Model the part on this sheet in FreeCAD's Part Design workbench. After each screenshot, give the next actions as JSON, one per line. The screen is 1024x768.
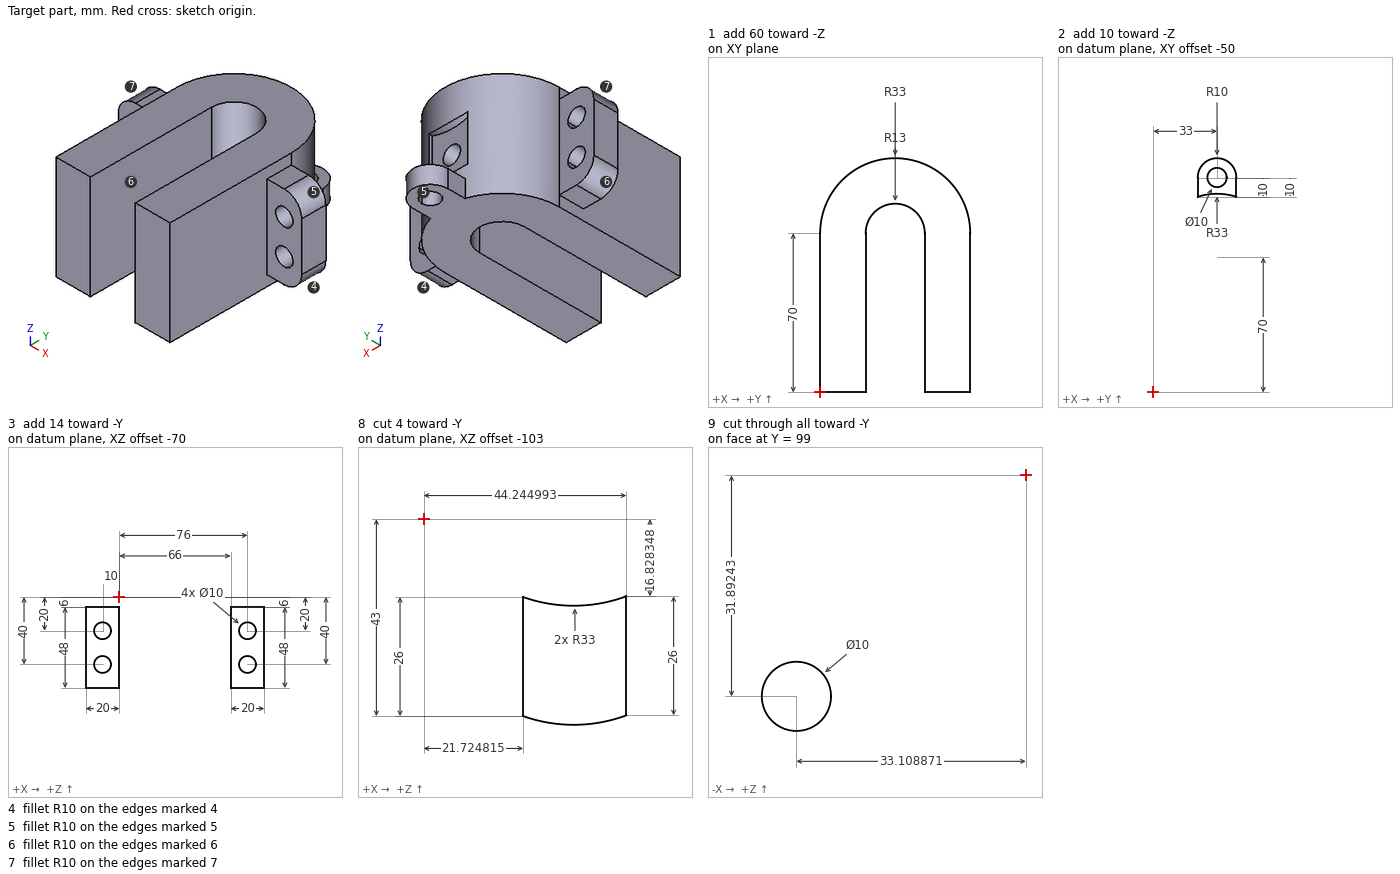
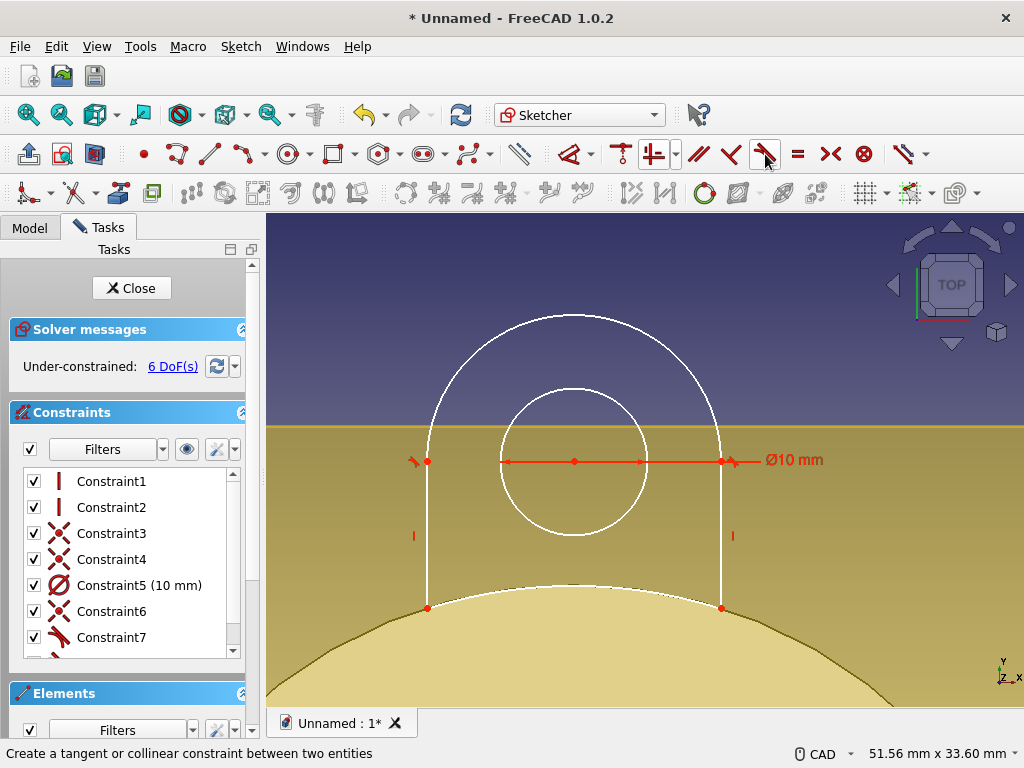
{"action": "left_click", "coordinate": [634, 590]}
{"action": "left_click", "coordinate": [638, 558]}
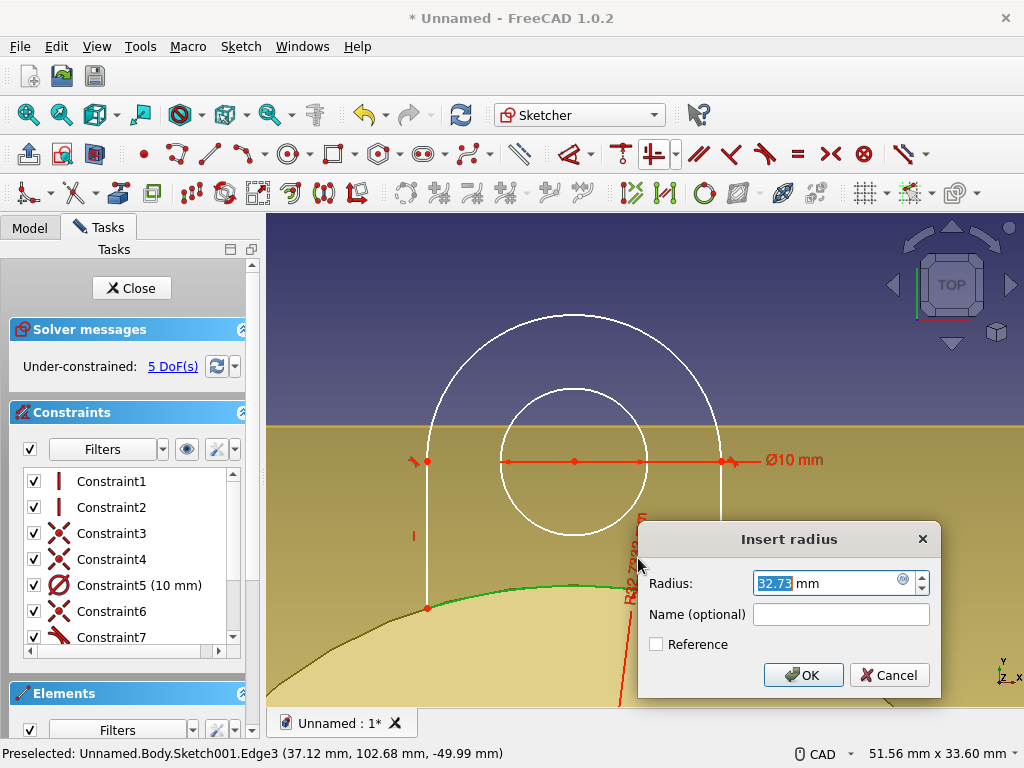
{"action": "type", "text": "33"}
{"action": "key", "text": "Return"}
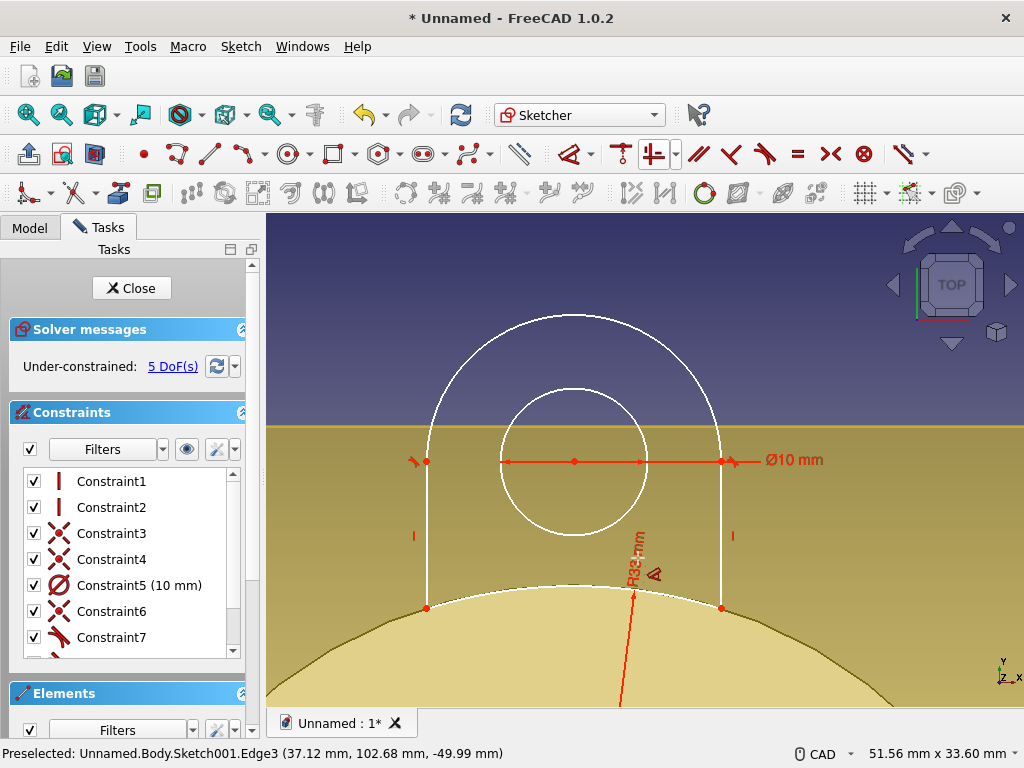
{"action": "left_click", "coordinate": [660, 343]}
{"action": "left_click", "coordinate": [679, 317]}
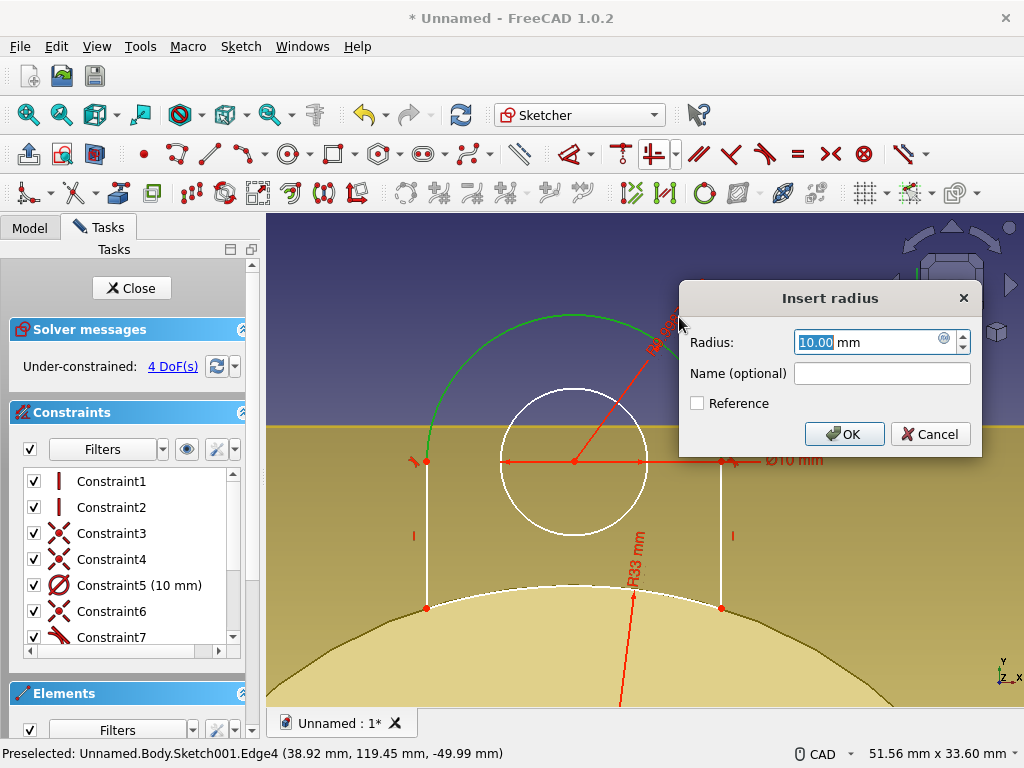
{"action": "type", "text": "10"}
{"action": "key", "text": "Return"}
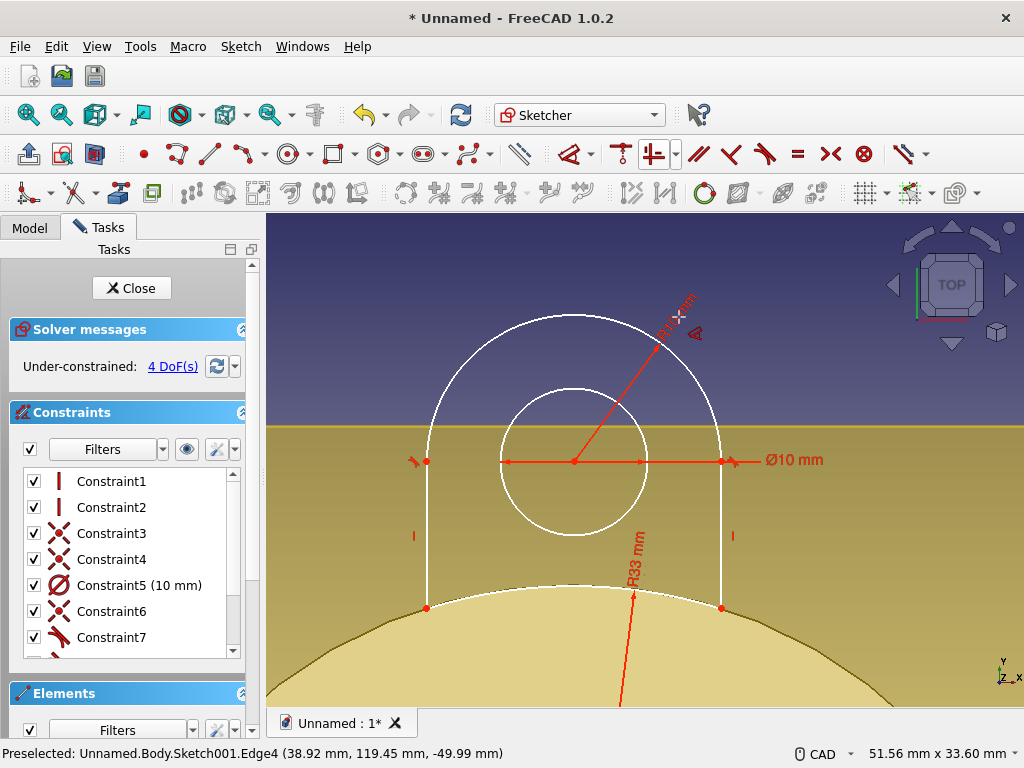
{"action": "left_click", "coordinate": [721, 506]}
{"action": "left_click", "coordinate": [755, 535]}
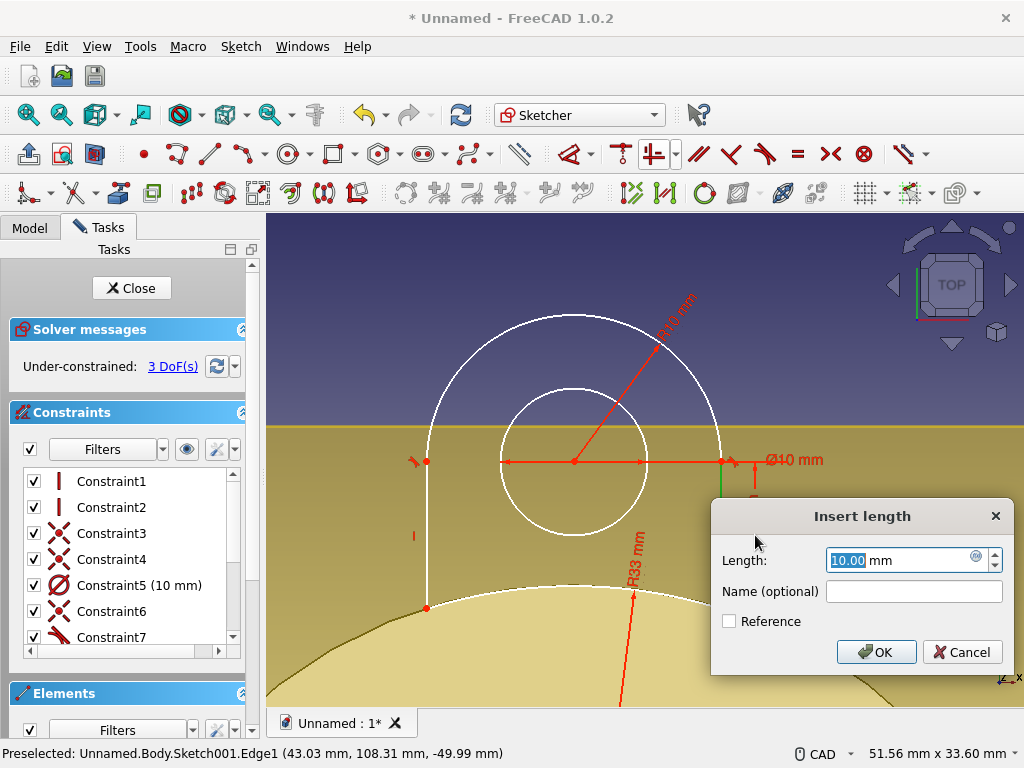
{"action": "type", "text": "10"}
{"action": "key", "text": "Return"}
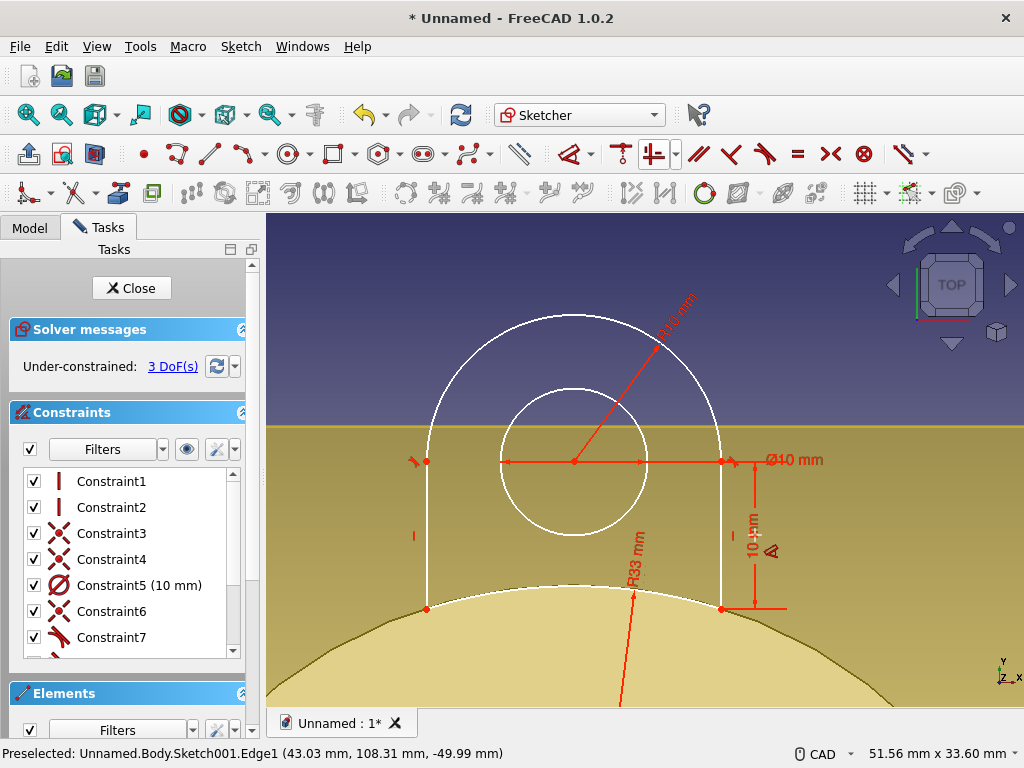
{"action": "left_click", "coordinate": [427, 565]}
{"action": "left_click", "coordinate": [393, 536]}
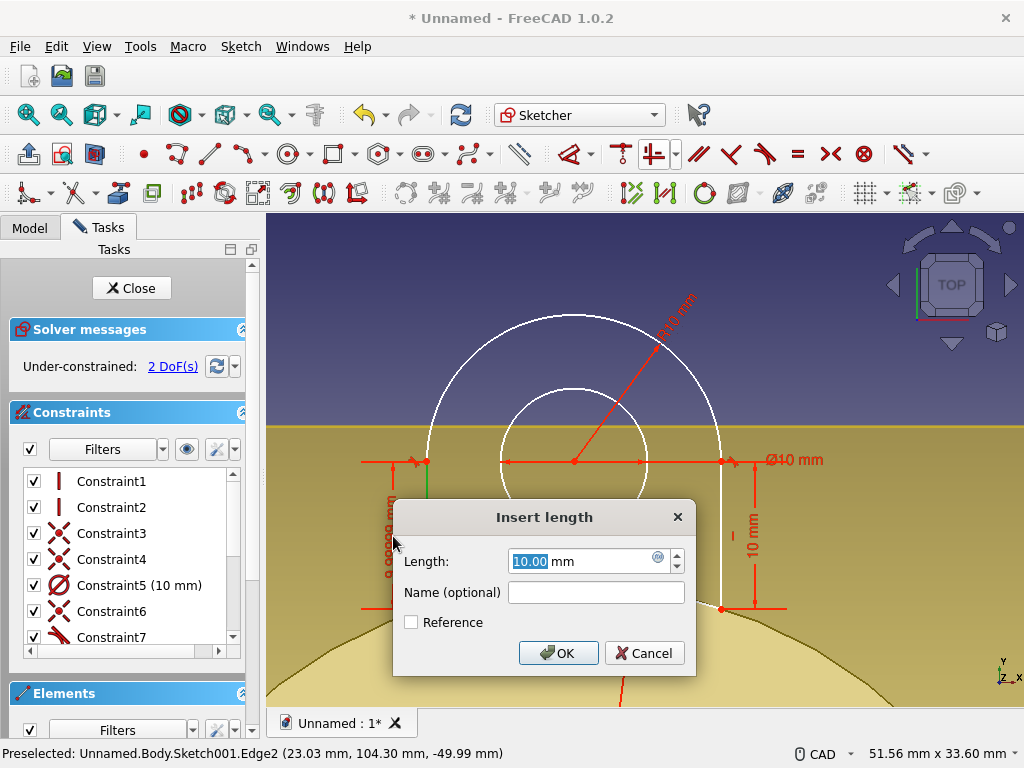
{"action": "type", "text": "10"}
{"action": "key", "text": "Return"}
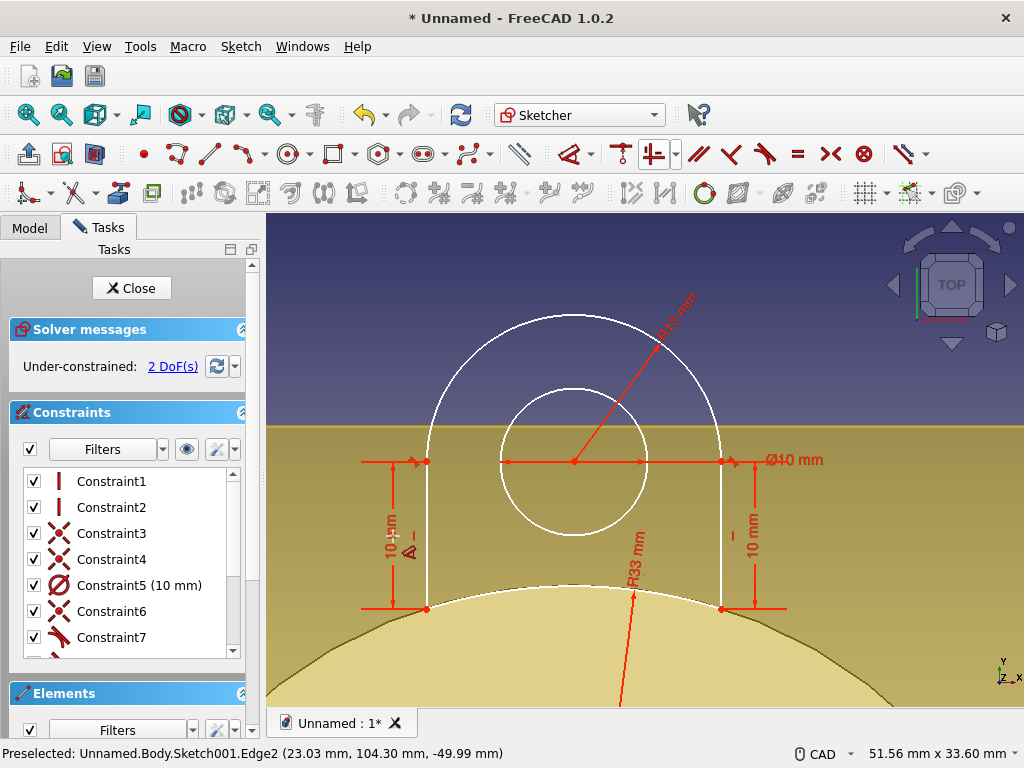
{"action": "left_click", "coordinate": [574, 462]}
{"action": "left_click", "coordinate": [370, 428]}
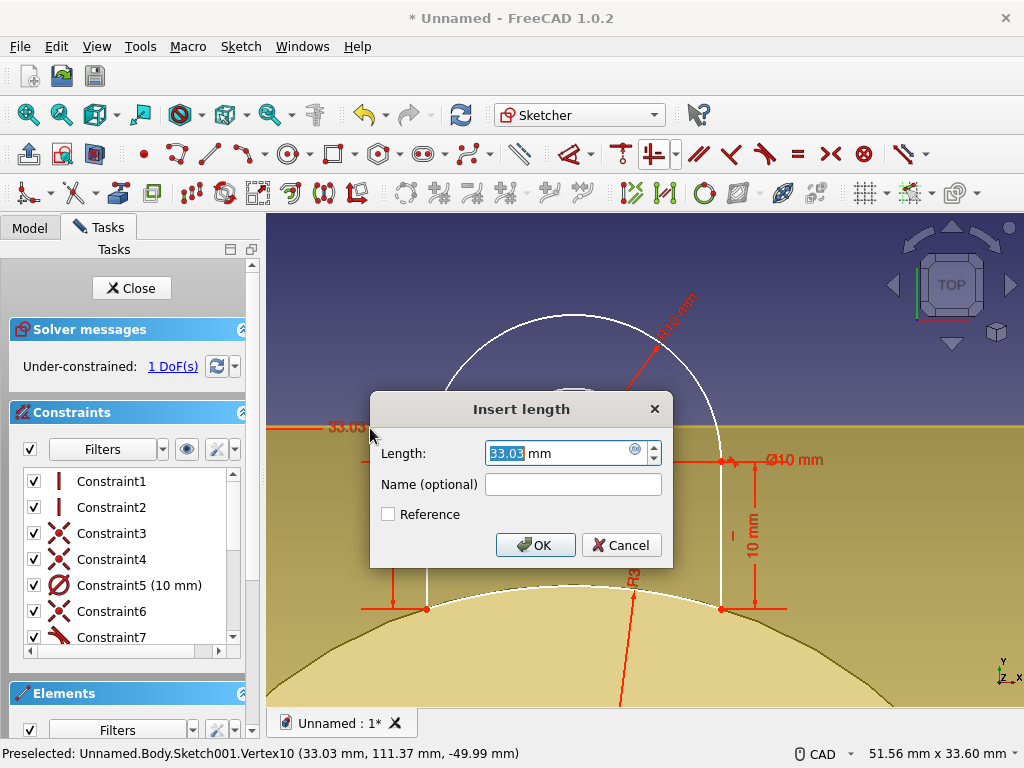
{"action": "type", "text": "33"}
{"action": "key", "text": "Return"}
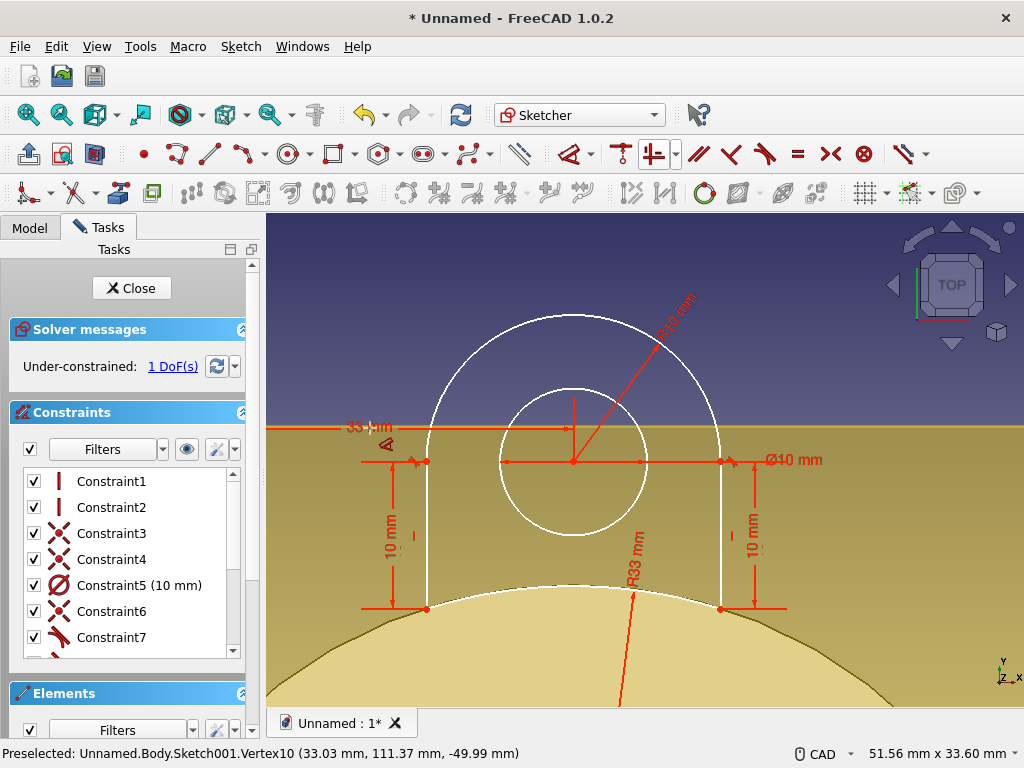
{"action": "scroll", "coordinate": [579, 270], "scroll_direction": "down", "scroll_amount": 4}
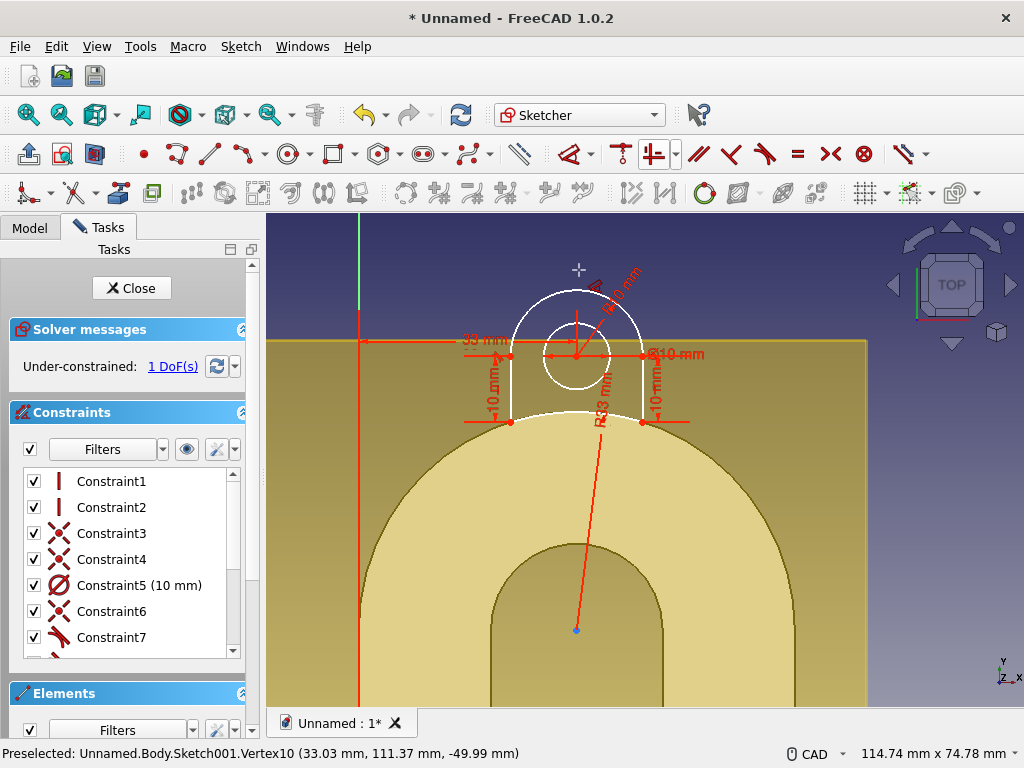
{"action": "left_click", "coordinate": [577, 630]}
{"action": "left_click", "coordinate": [325, 655]}